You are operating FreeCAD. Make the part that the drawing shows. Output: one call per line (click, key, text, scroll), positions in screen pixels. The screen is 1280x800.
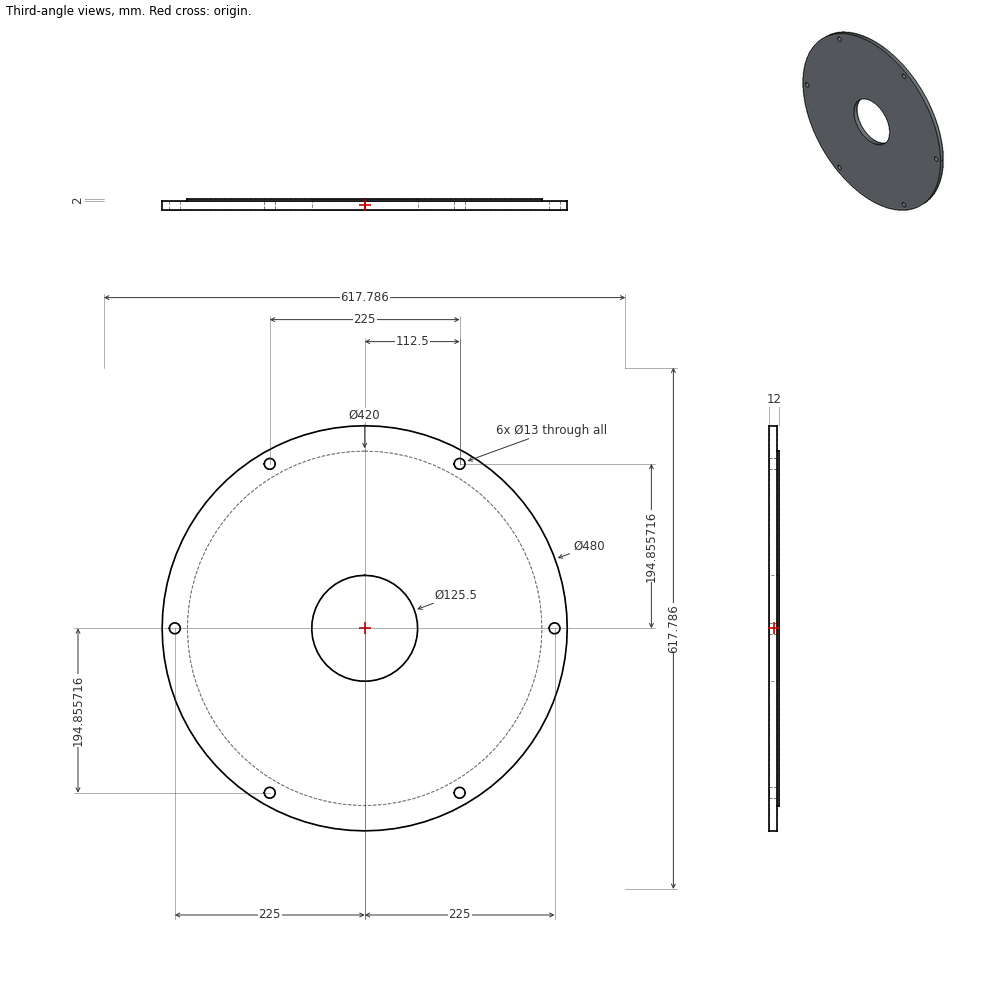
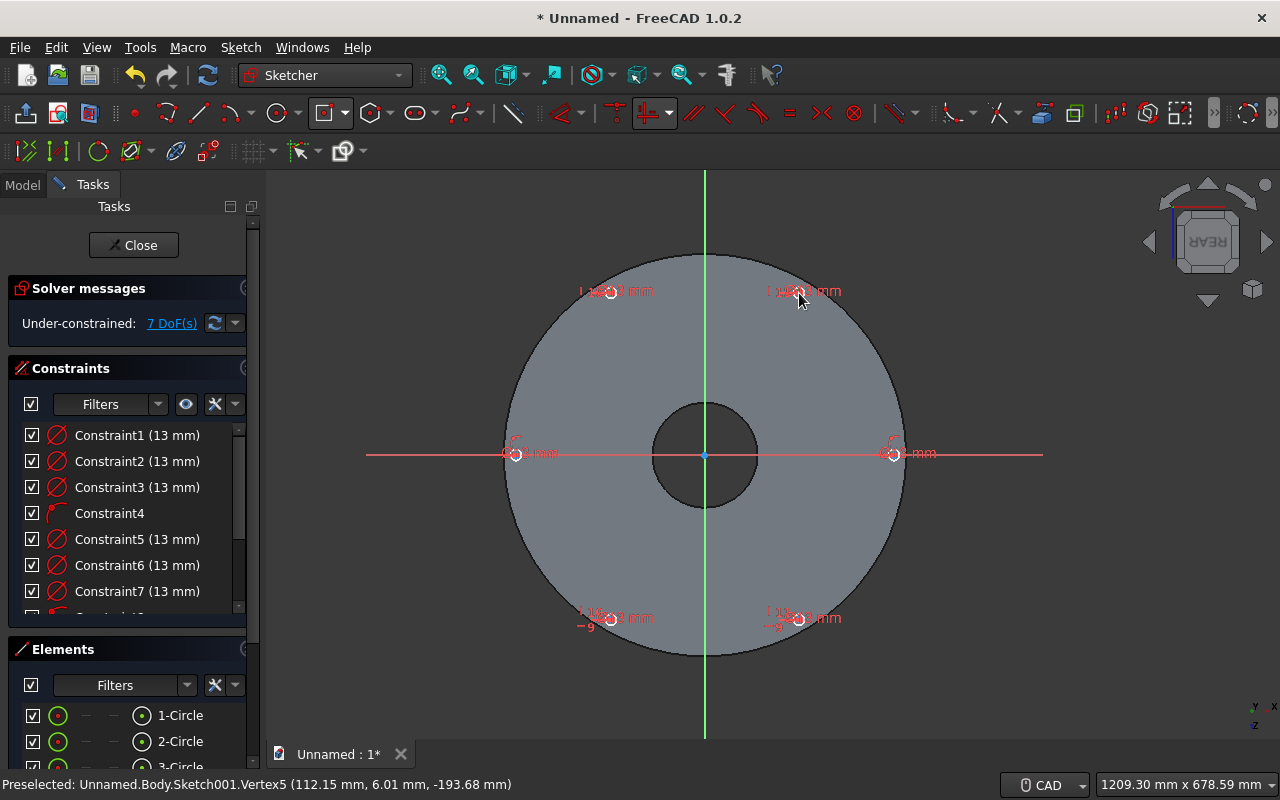
key(h)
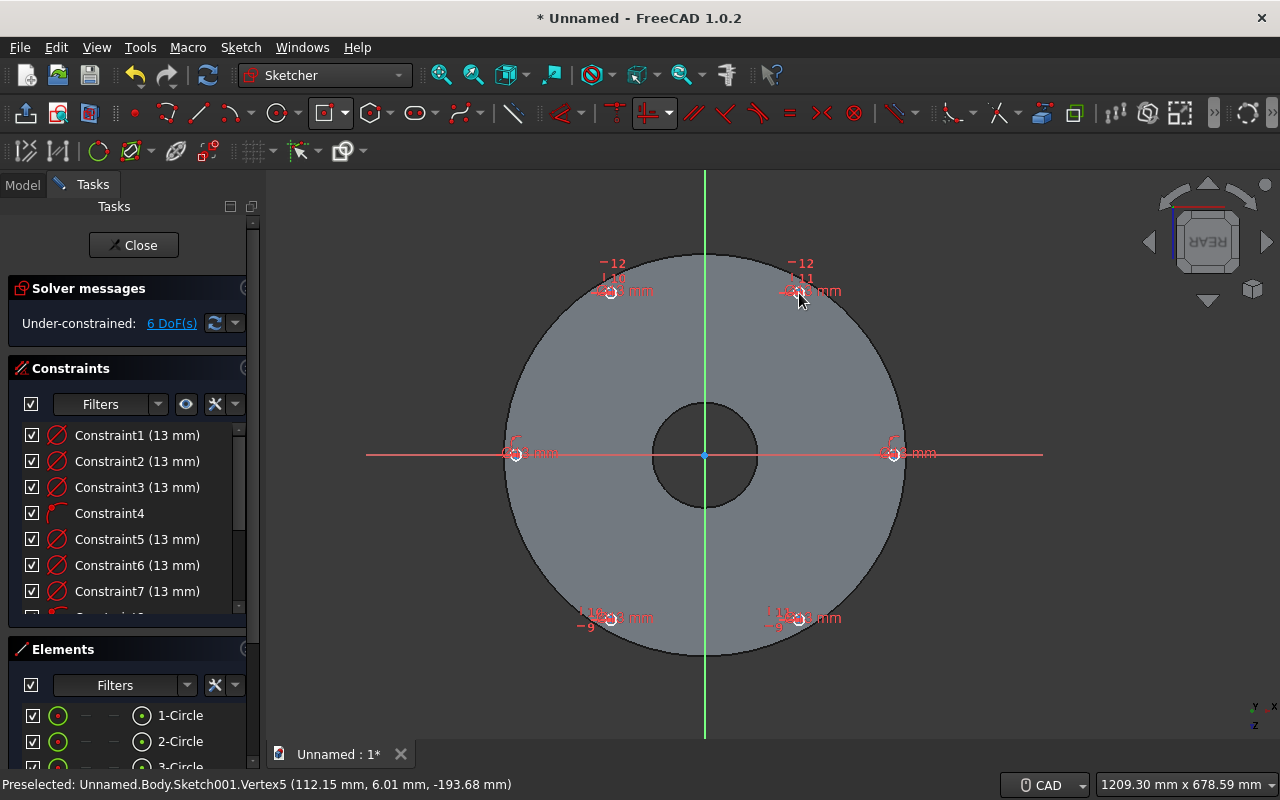
click(560, 114)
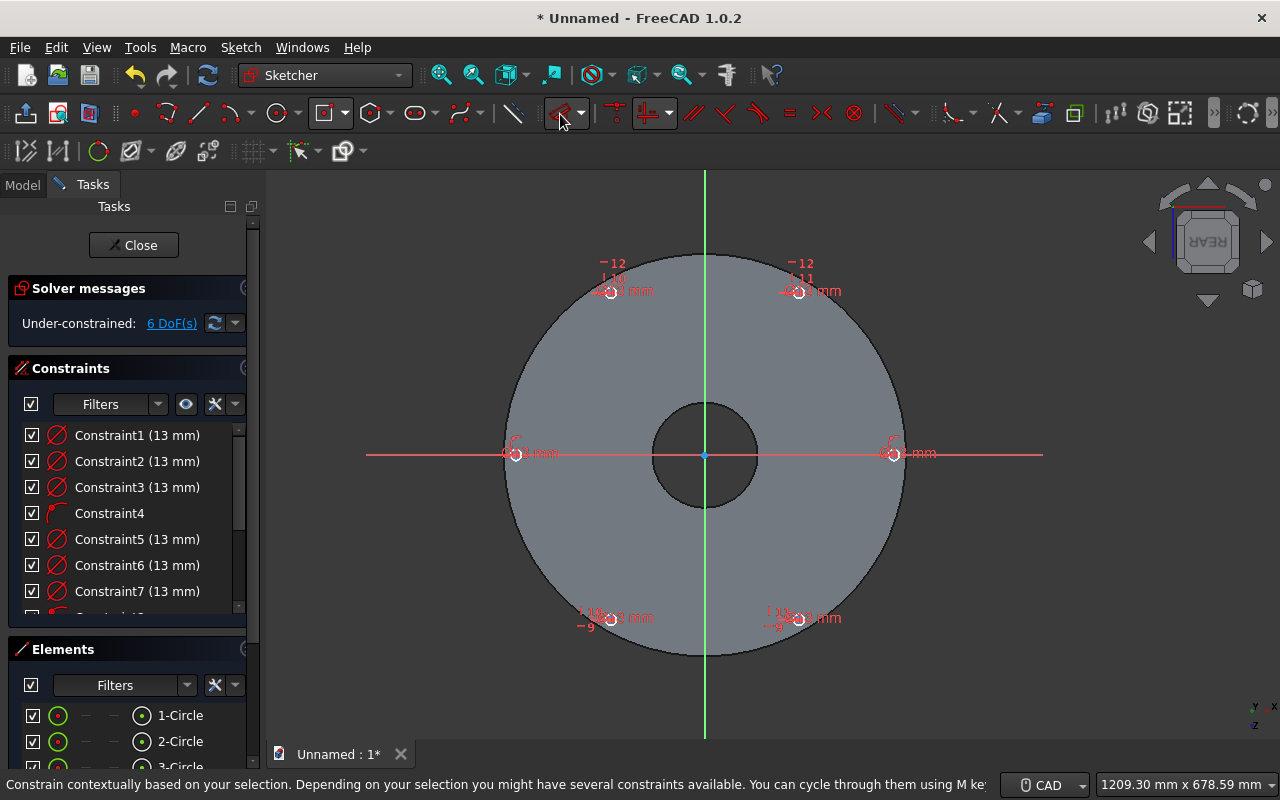
click(516, 455)
click(610, 489)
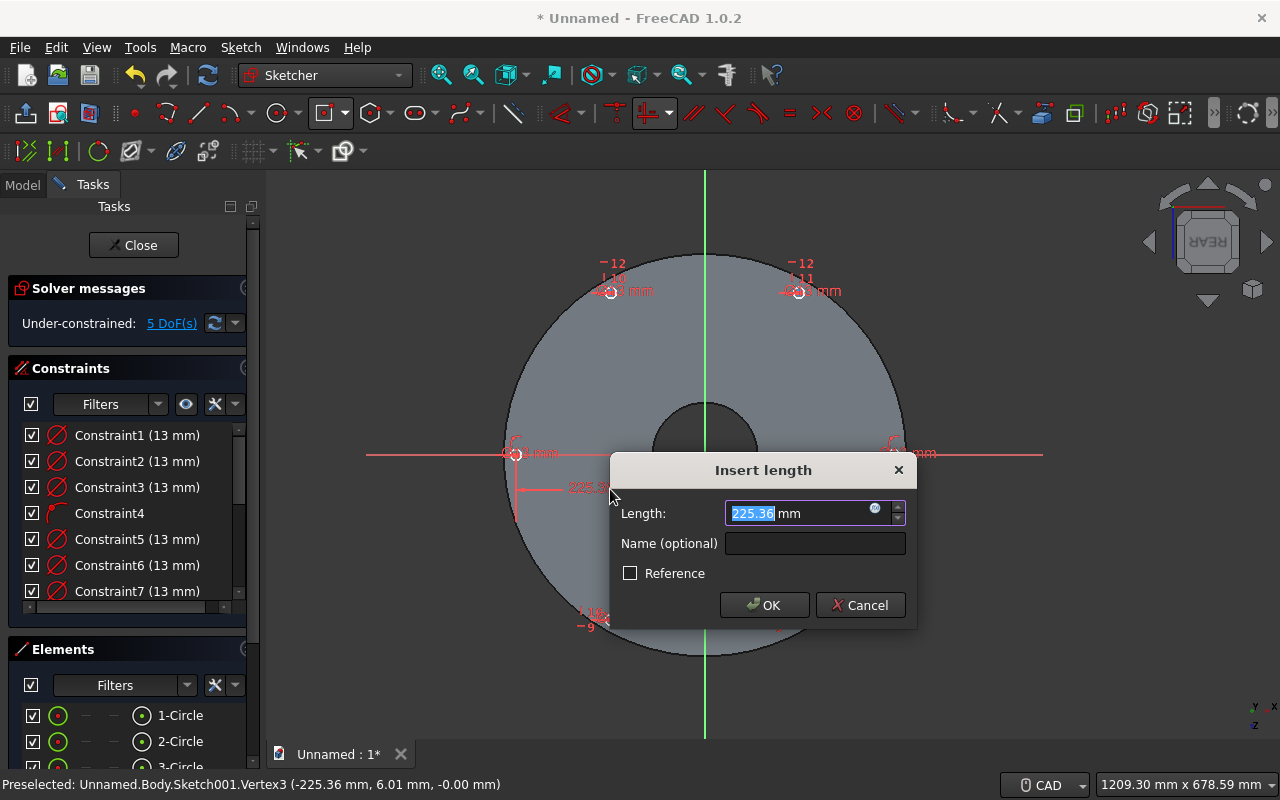
text(225)
key(Return)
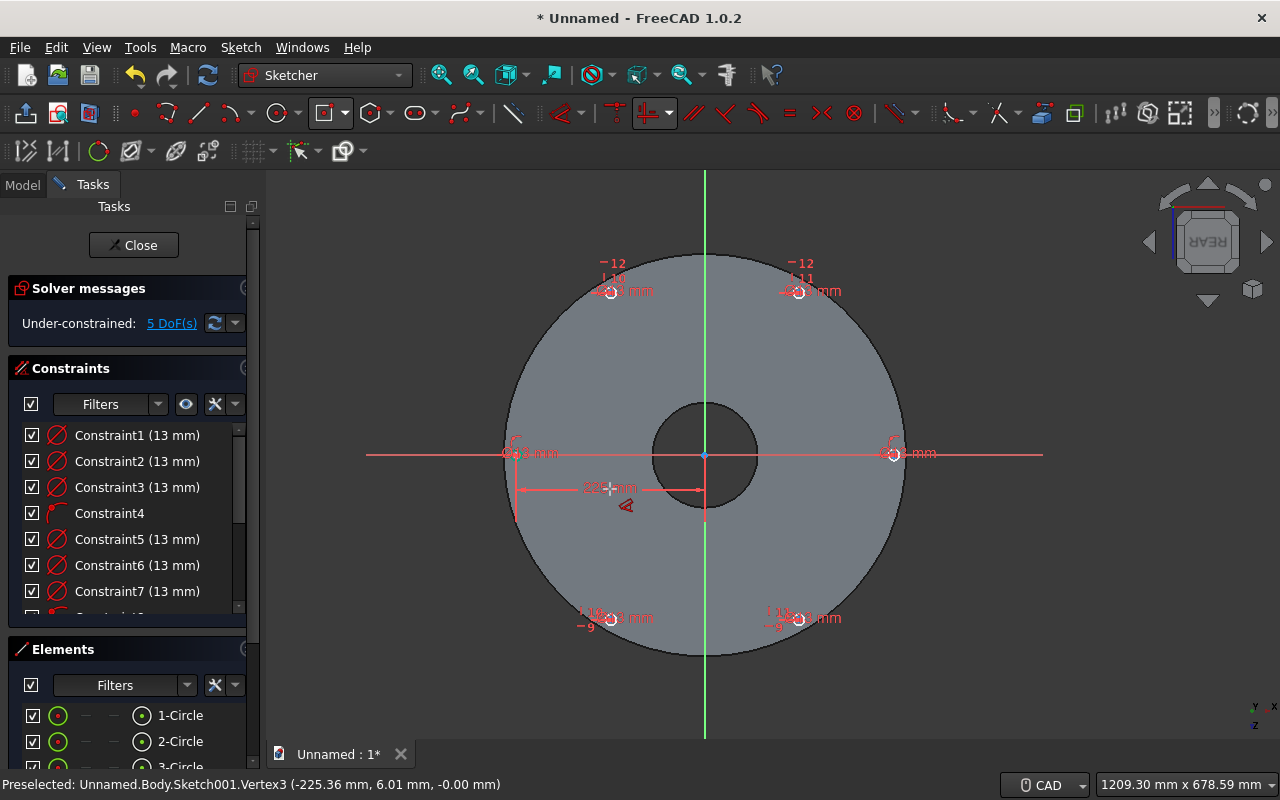
click(894, 455)
click(799, 489)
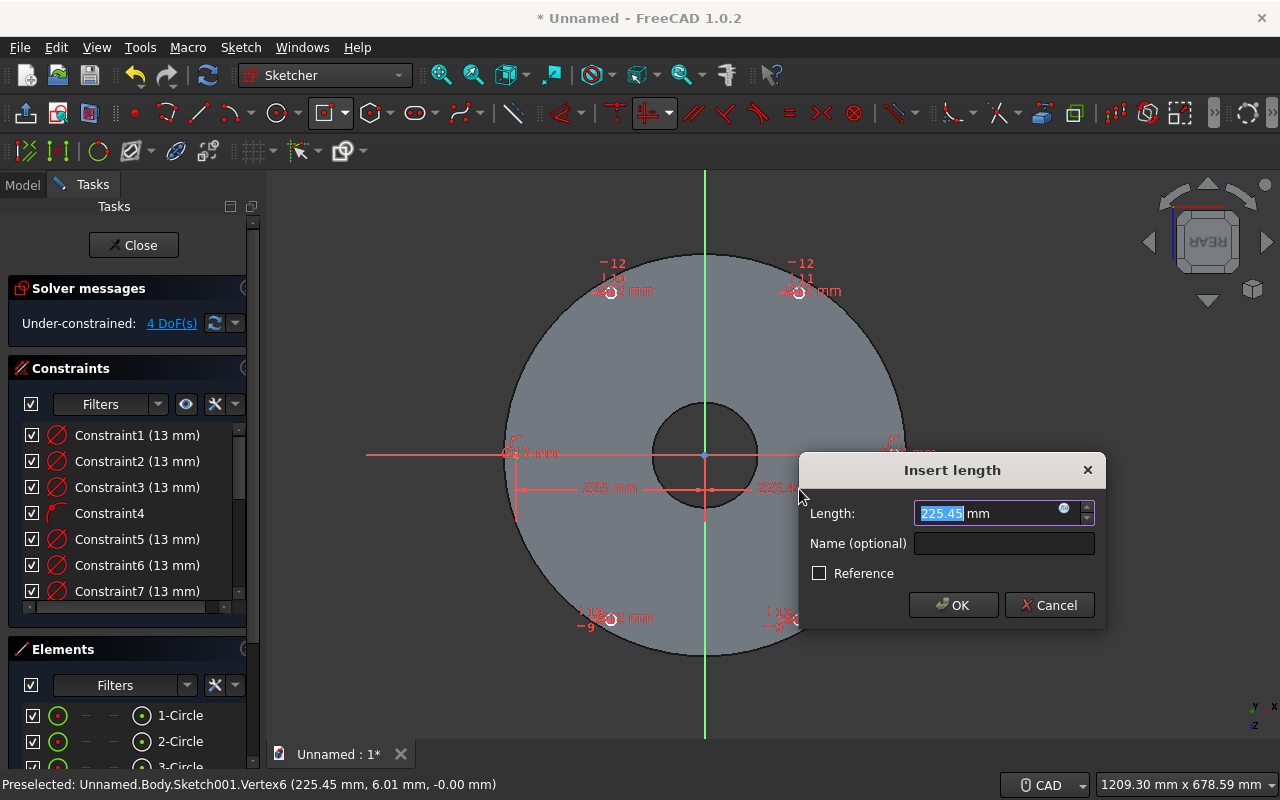
text(225)
key(Return)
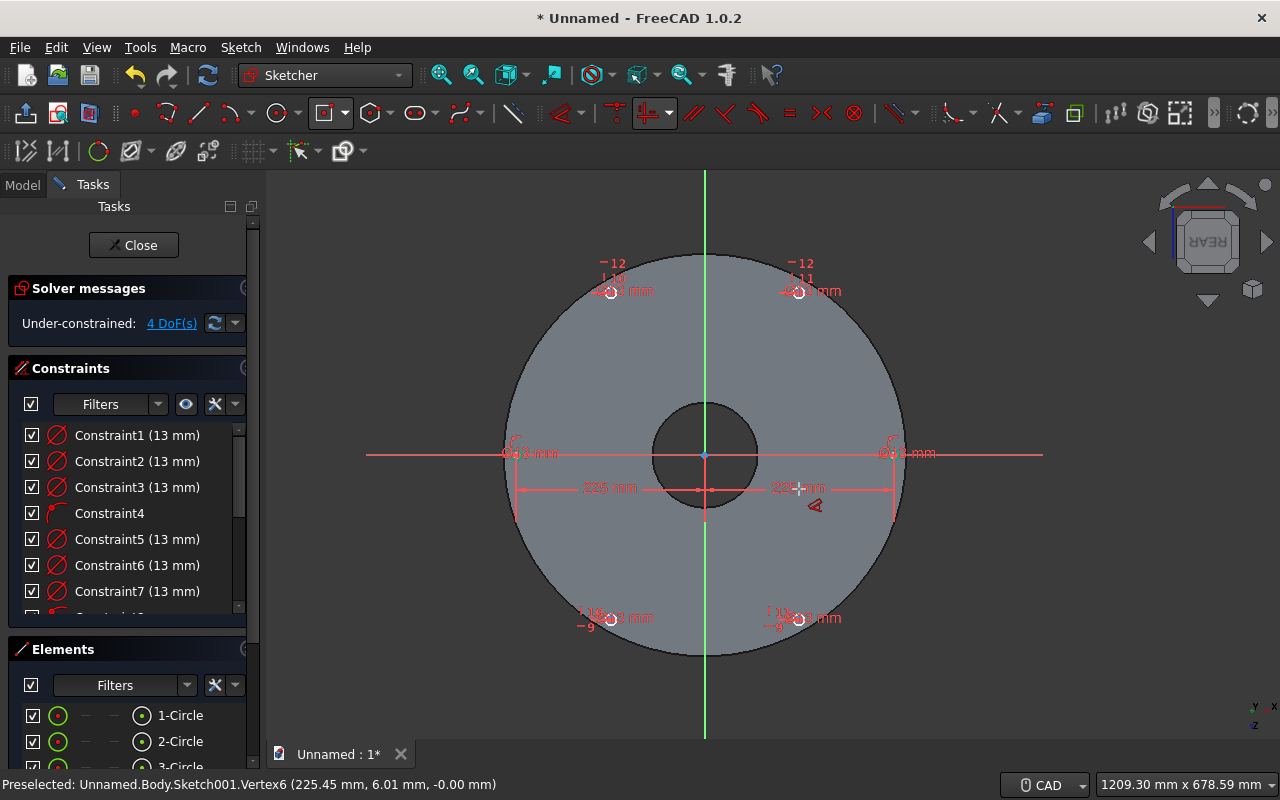
click(799, 620)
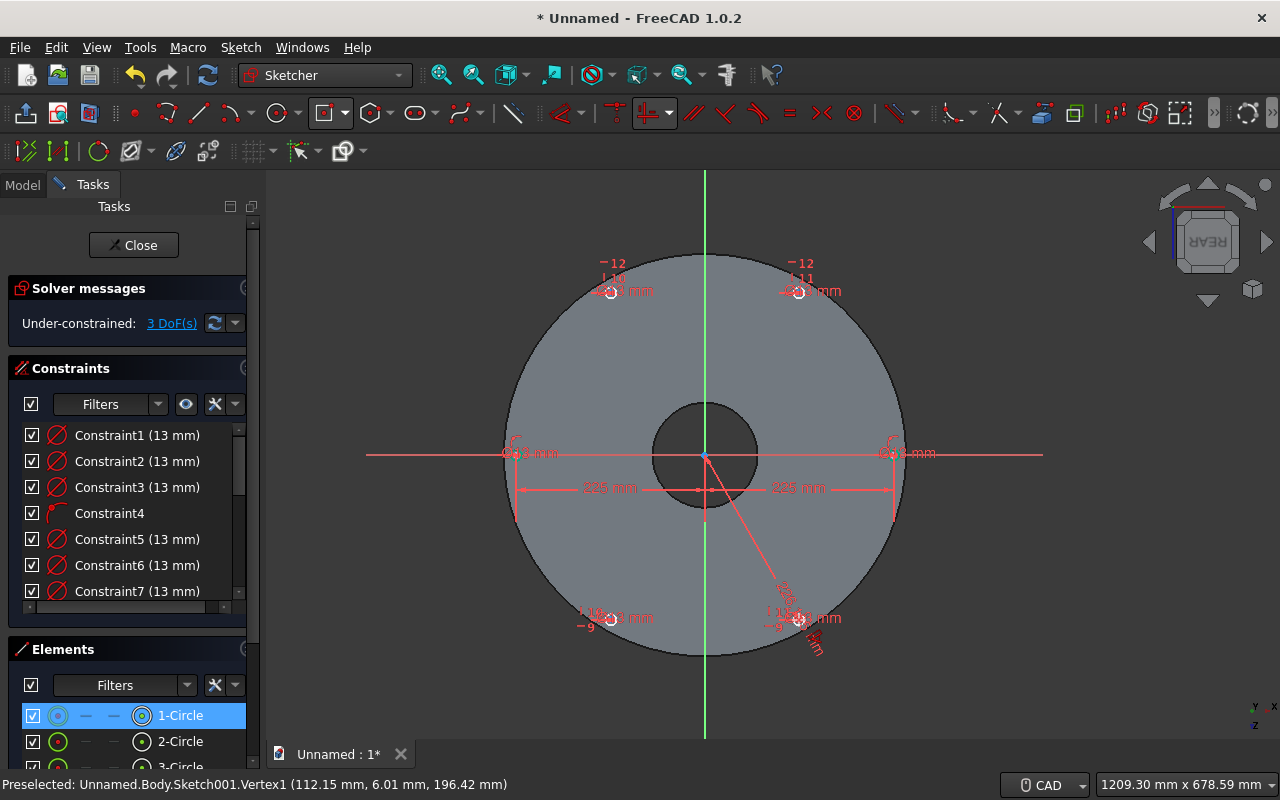
click(611, 620)
click(662, 654)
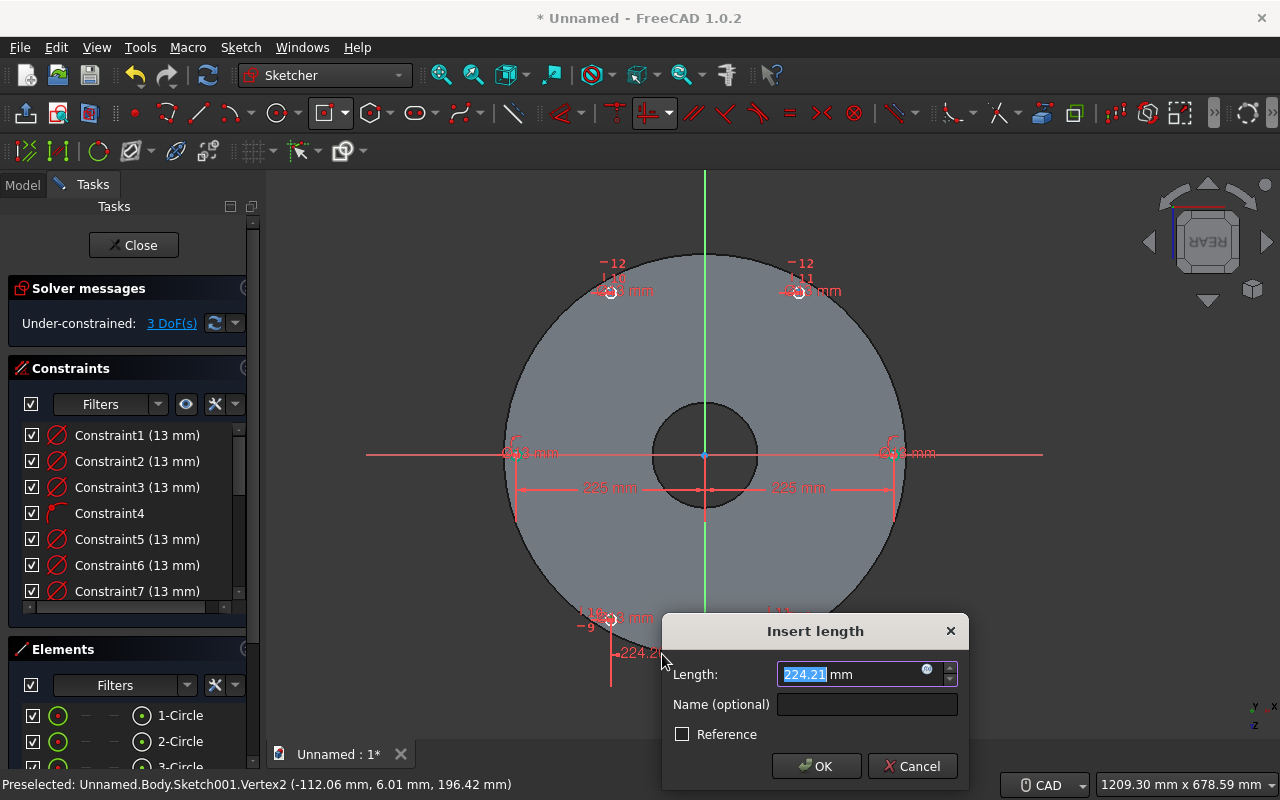
text(225)
key(Return)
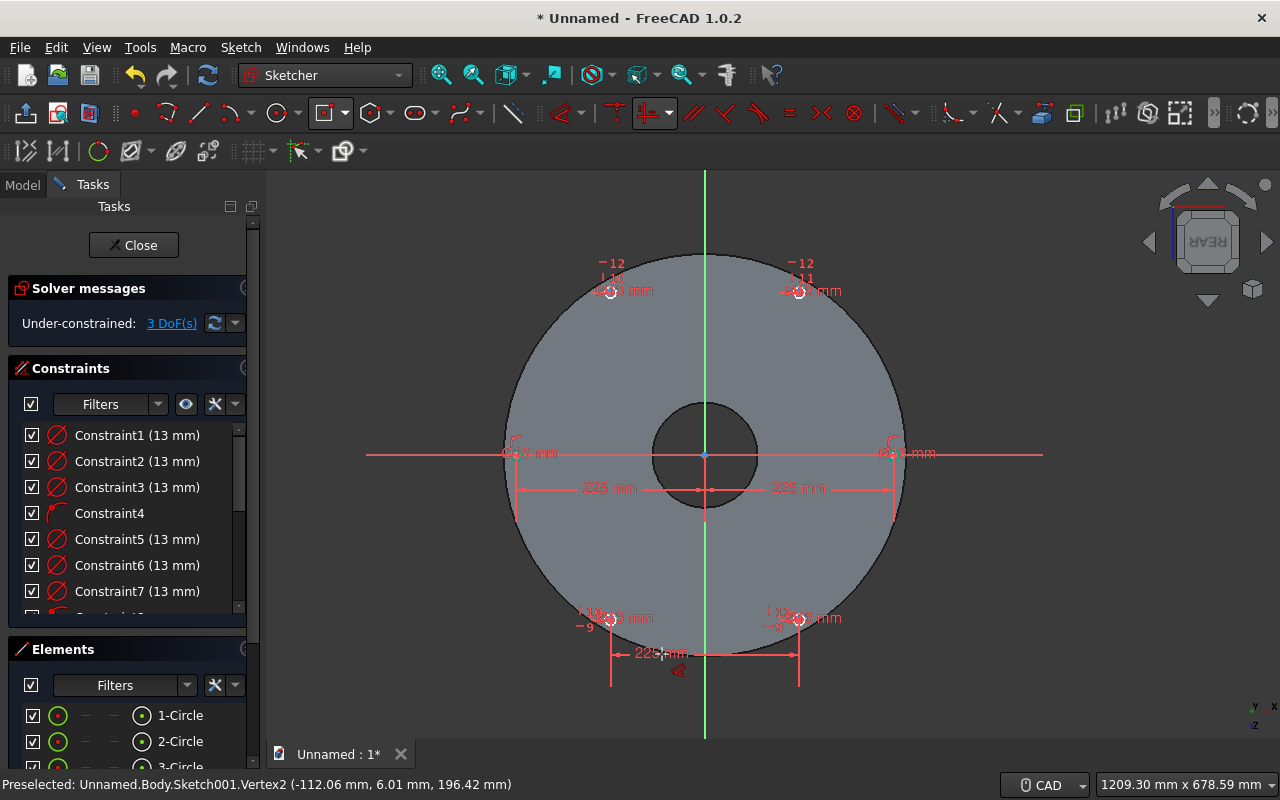
click(799, 620)
click(752, 654)